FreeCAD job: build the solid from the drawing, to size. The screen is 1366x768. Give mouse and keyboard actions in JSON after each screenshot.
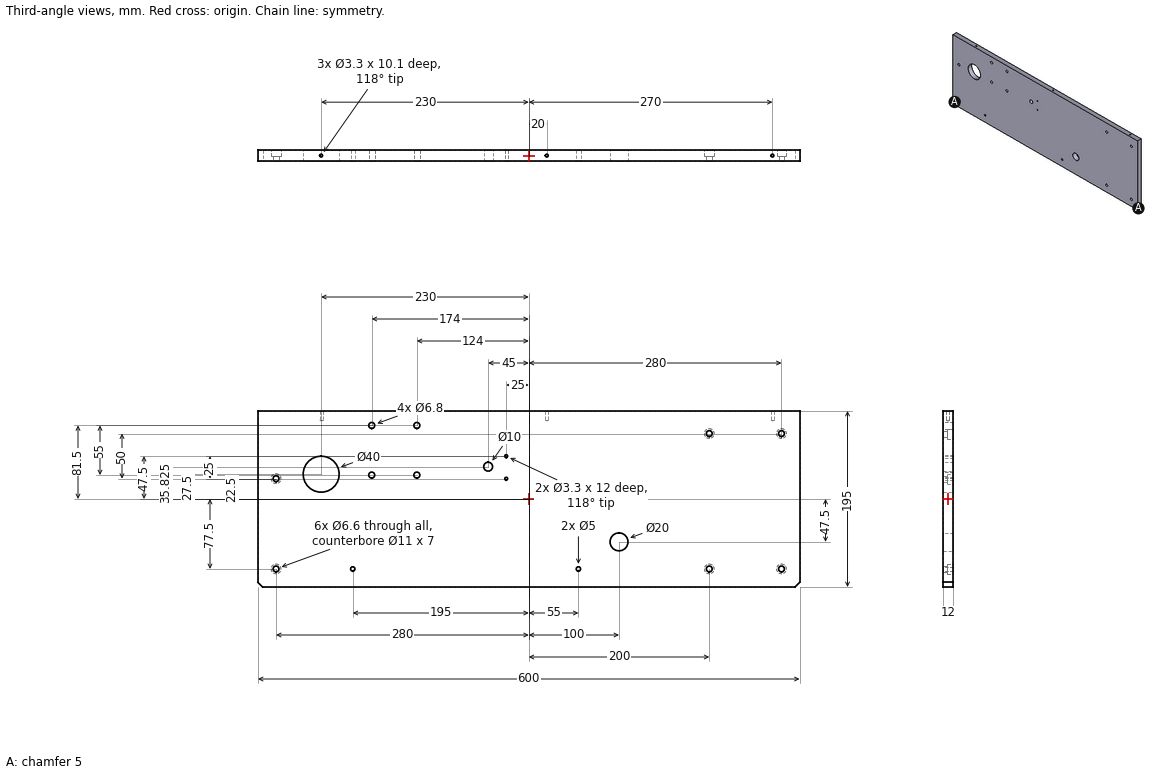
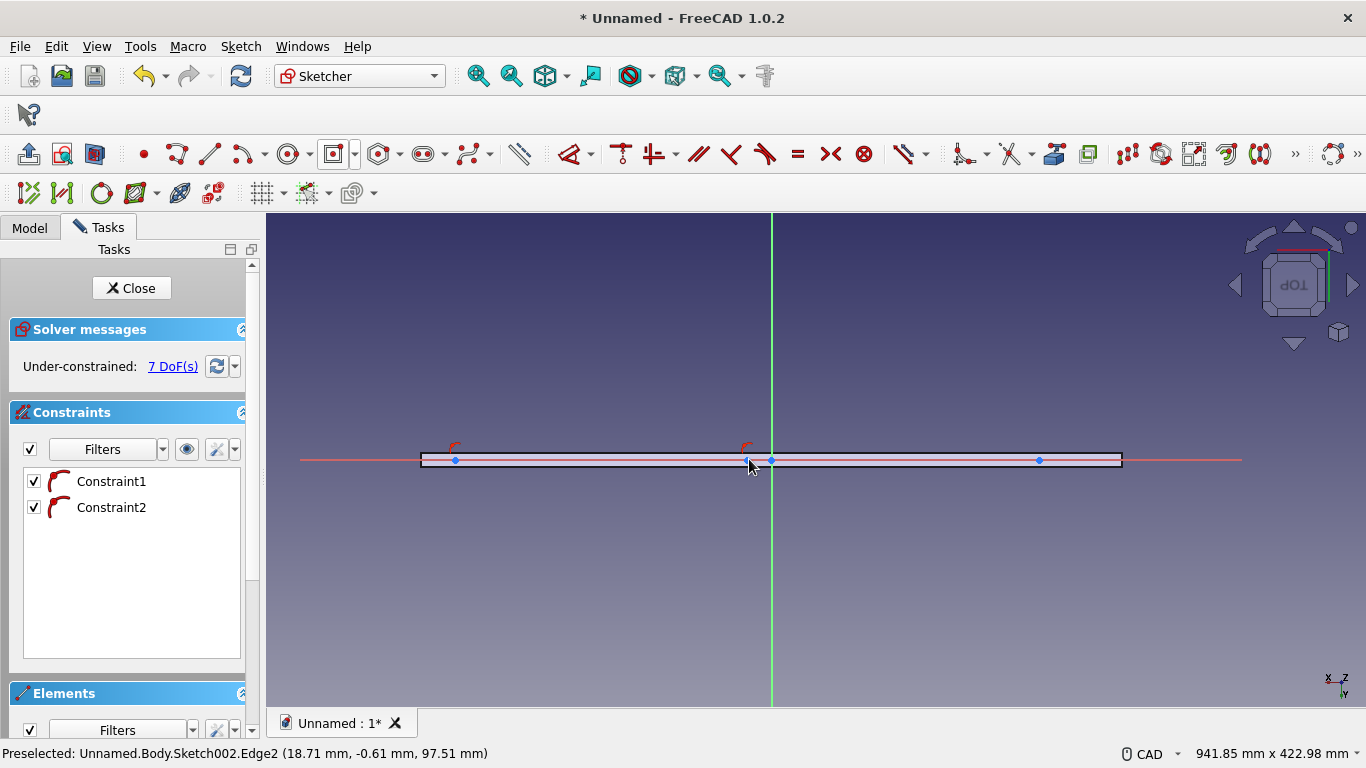
{"action": "scroll", "coordinate": [457, 459], "scroll_direction": "up", "scroll_amount": 12}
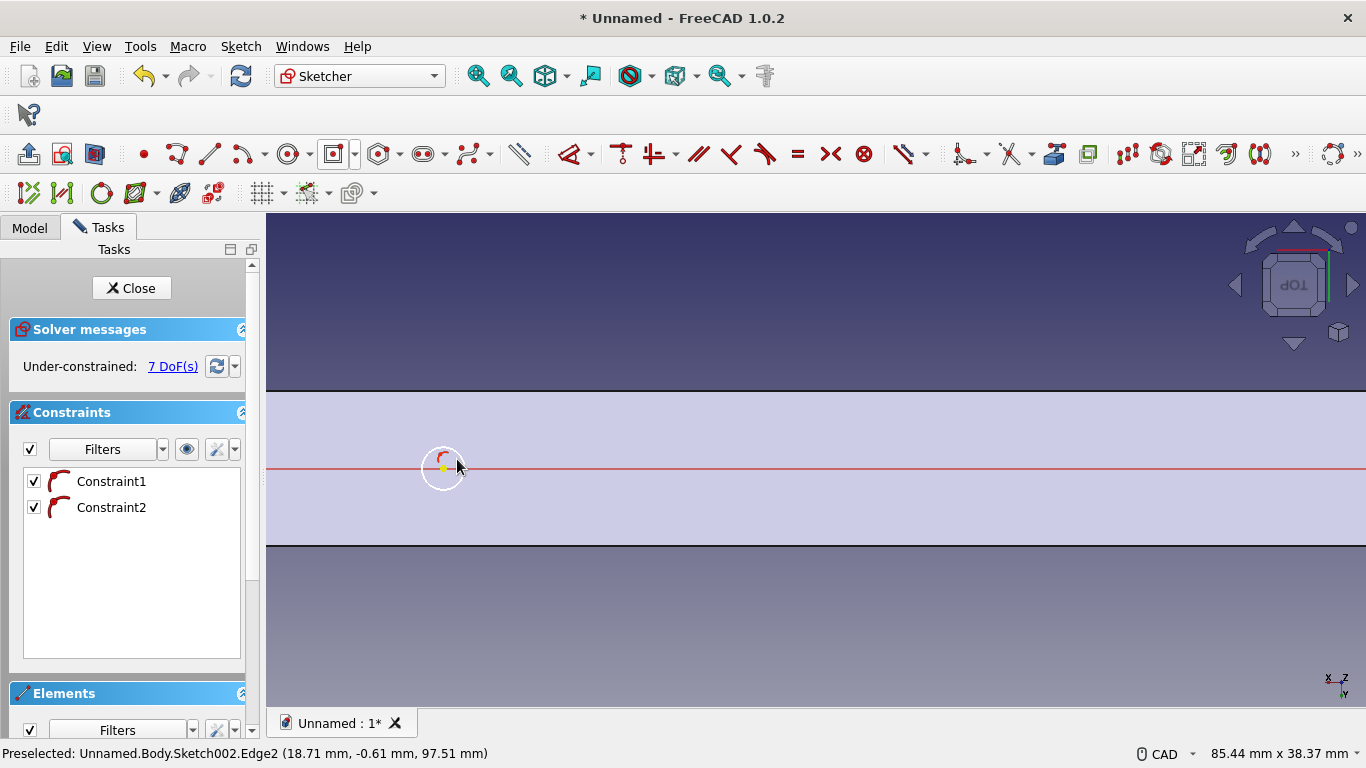
{"action": "left_click", "coordinate": [458, 454]}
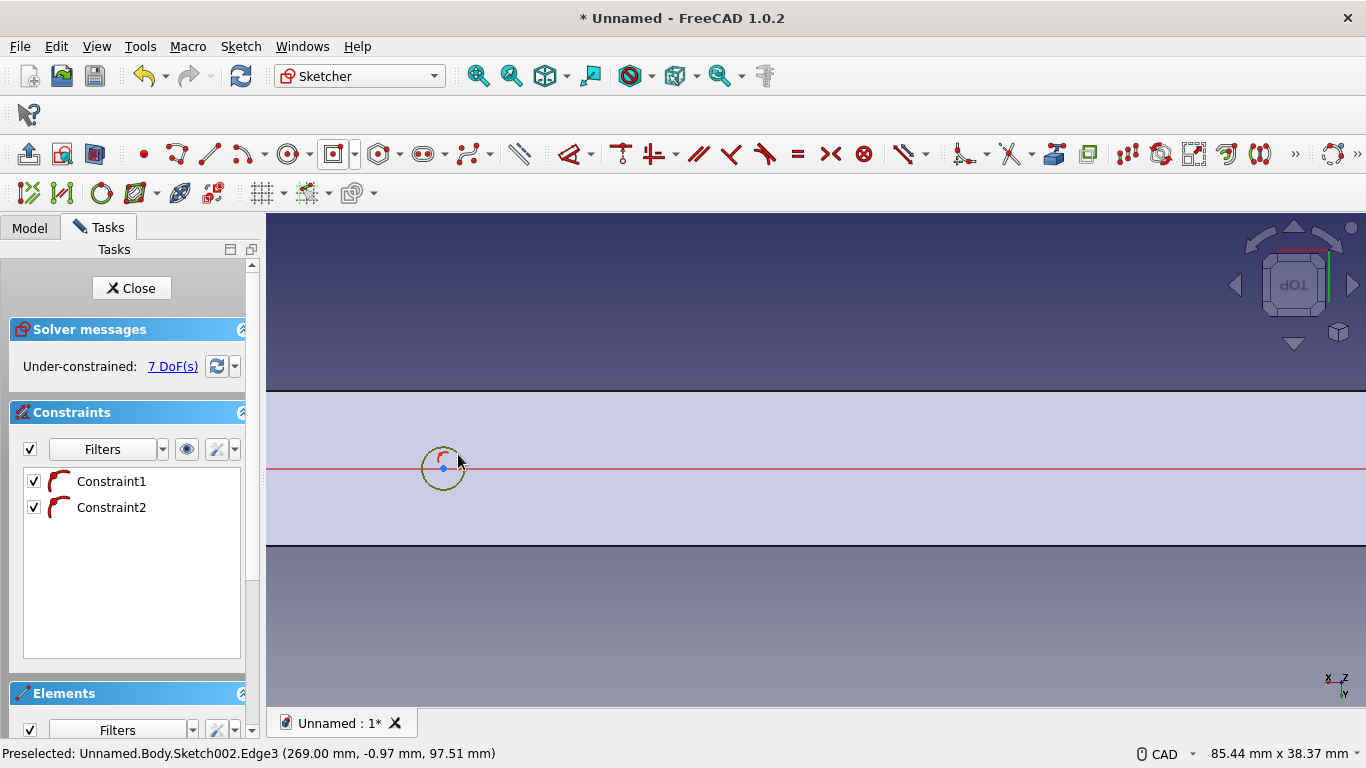
{"action": "left_click", "coordinate": [798, 154]}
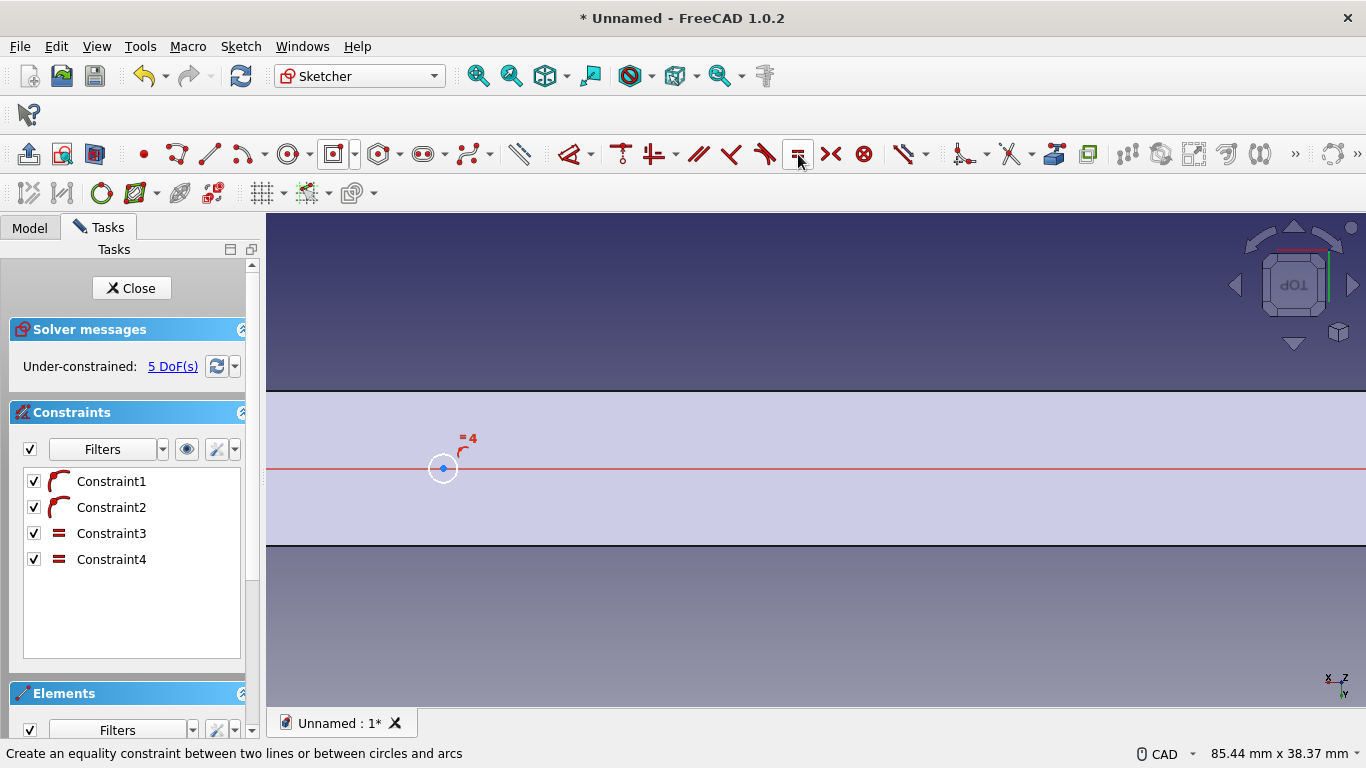
{"action": "scroll", "coordinate": [456, 459], "scroll_direction": "down", "scroll_amount": 12}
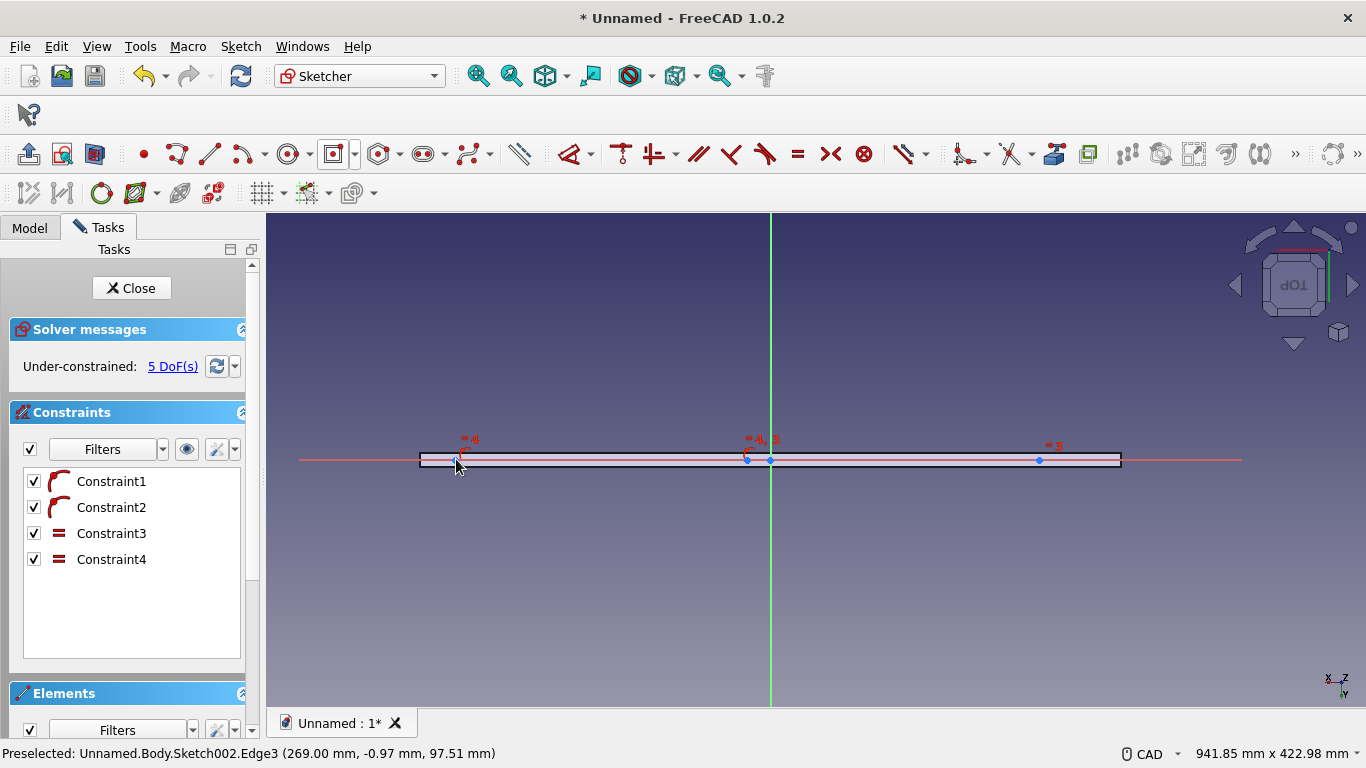
{"action": "left_click", "coordinate": [1039, 461]}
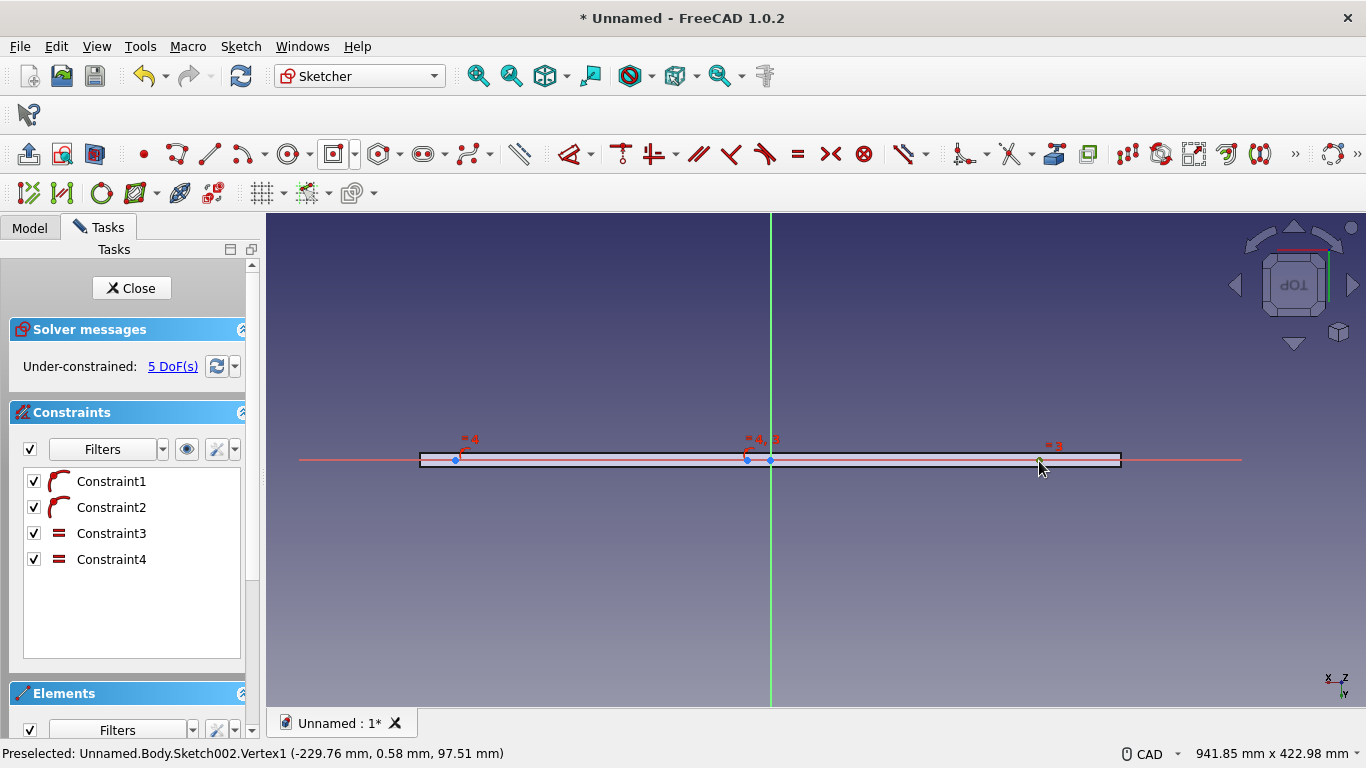
{"action": "left_click", "coordinate": [359, 460]}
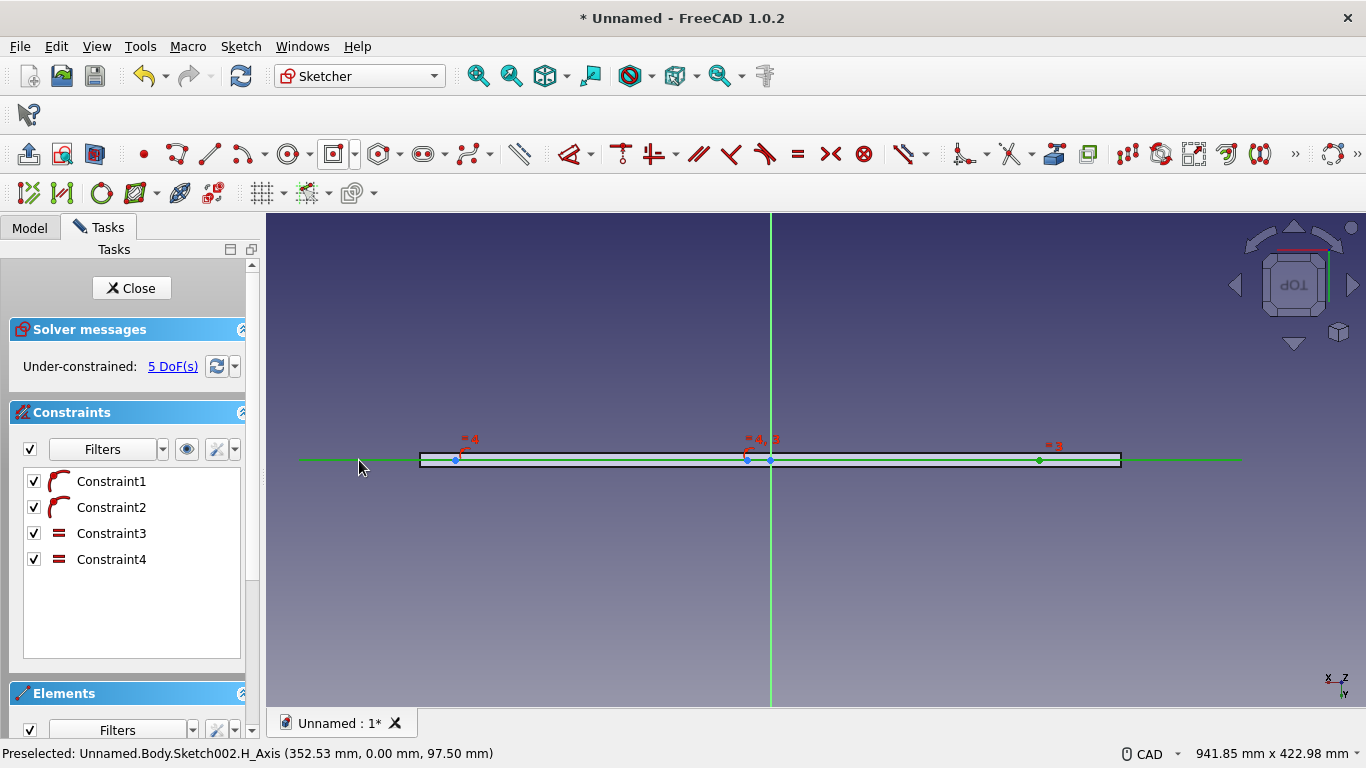
{"action": "key", "text": "c"}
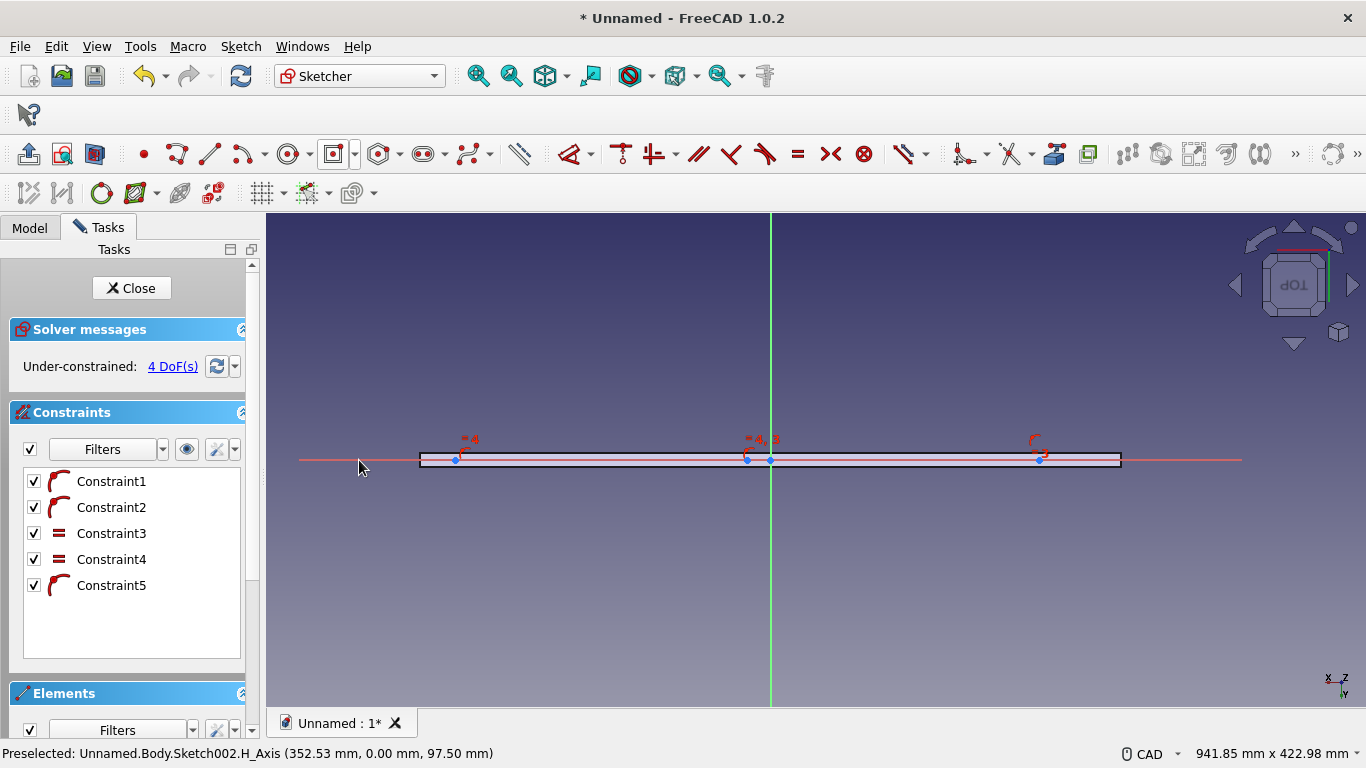
{"action": "key", "text": "d"}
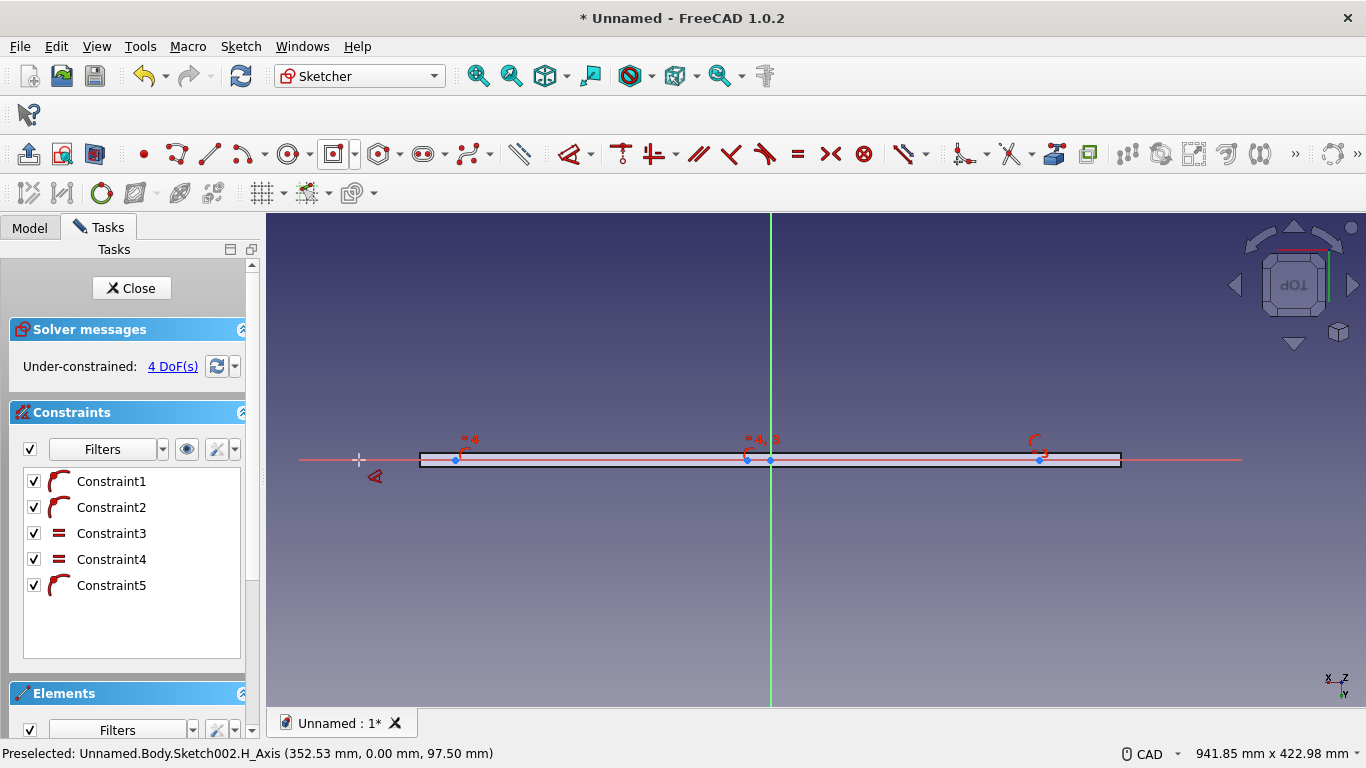
{"action": "scroll", "coordinate": [1039, 459], "scroll_direction": "up", "scroll_amount": 12}